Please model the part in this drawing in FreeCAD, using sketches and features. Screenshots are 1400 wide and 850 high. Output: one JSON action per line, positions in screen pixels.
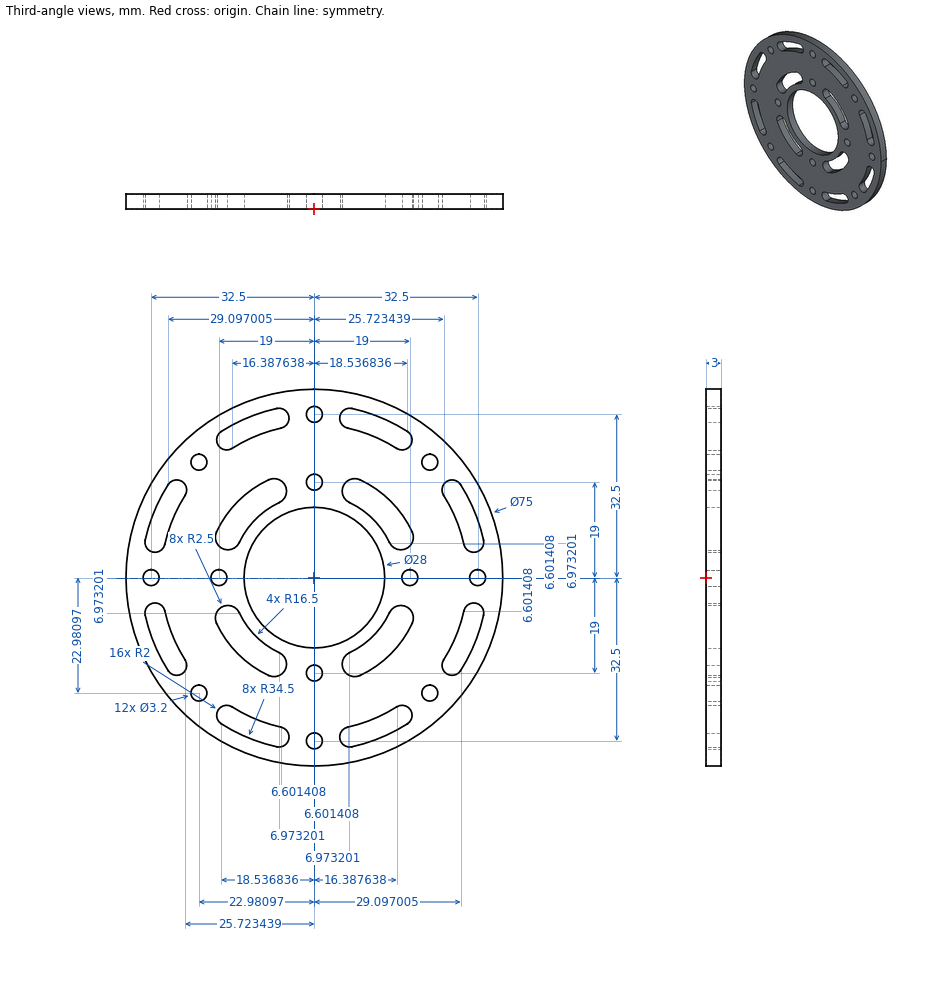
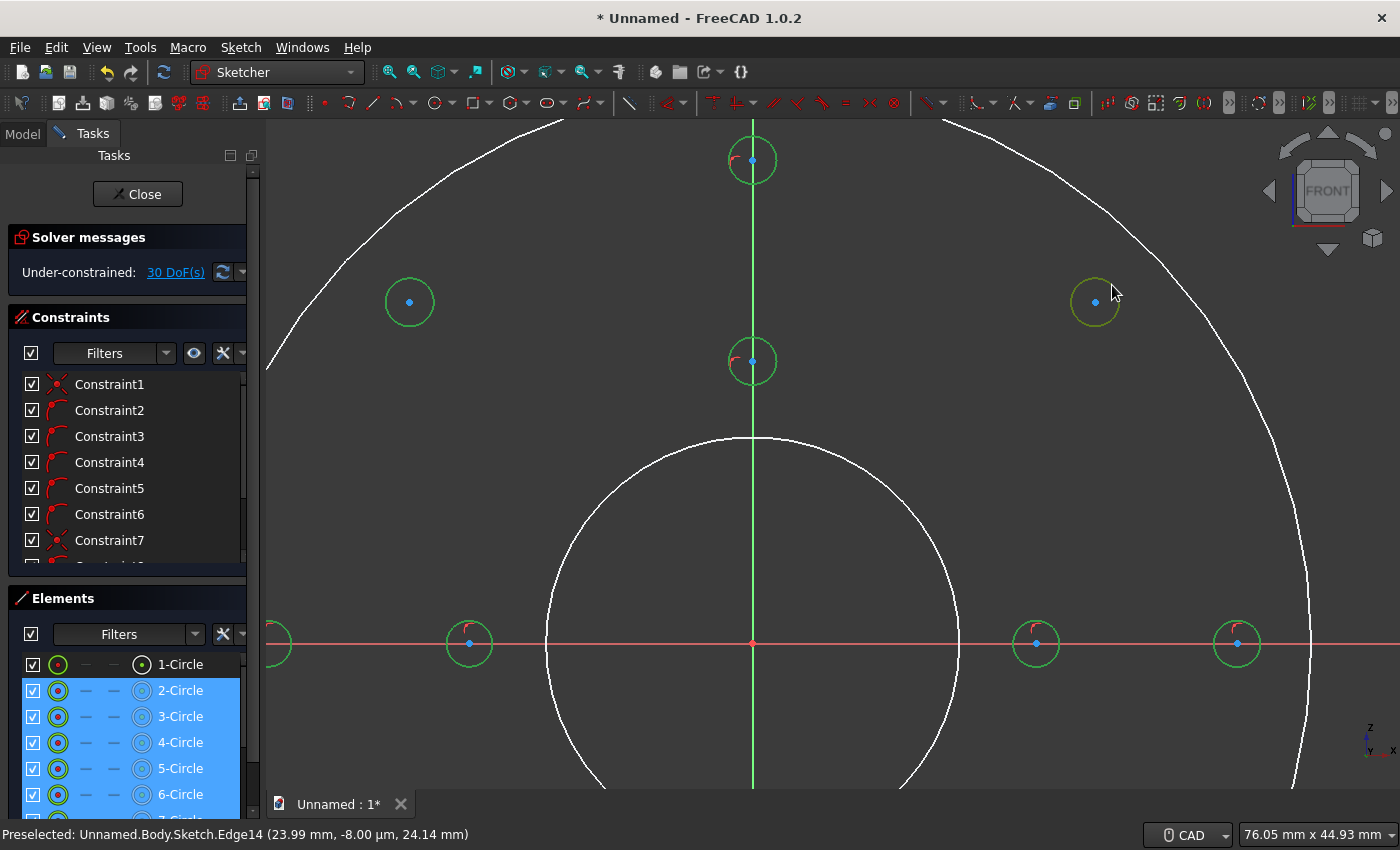
{"action": "left_click", "coordinate": [846, 104]}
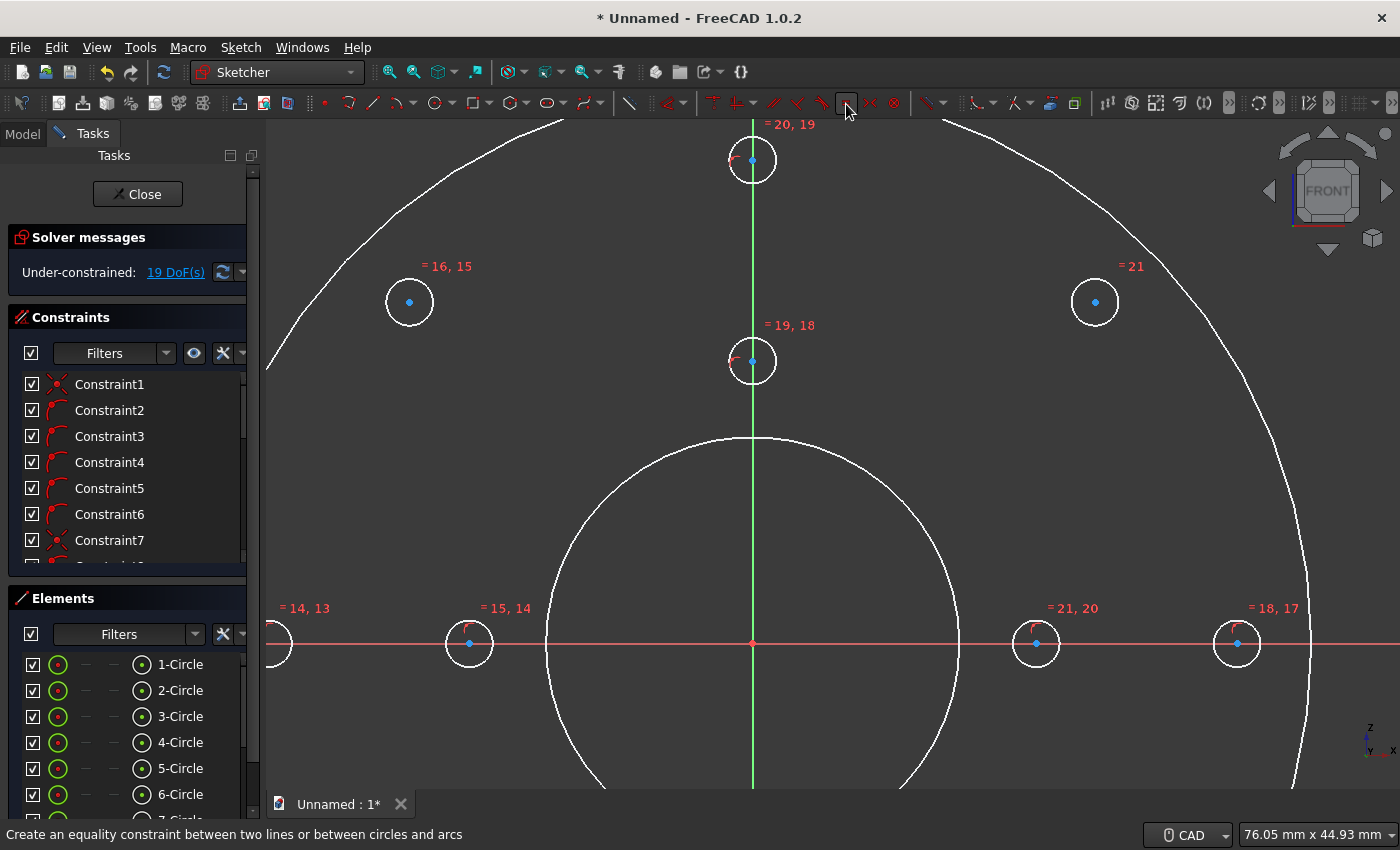
{"action": "scroll", "coordinate": [771, 344], "scroll_direction": "down", "scroll_amount": 5}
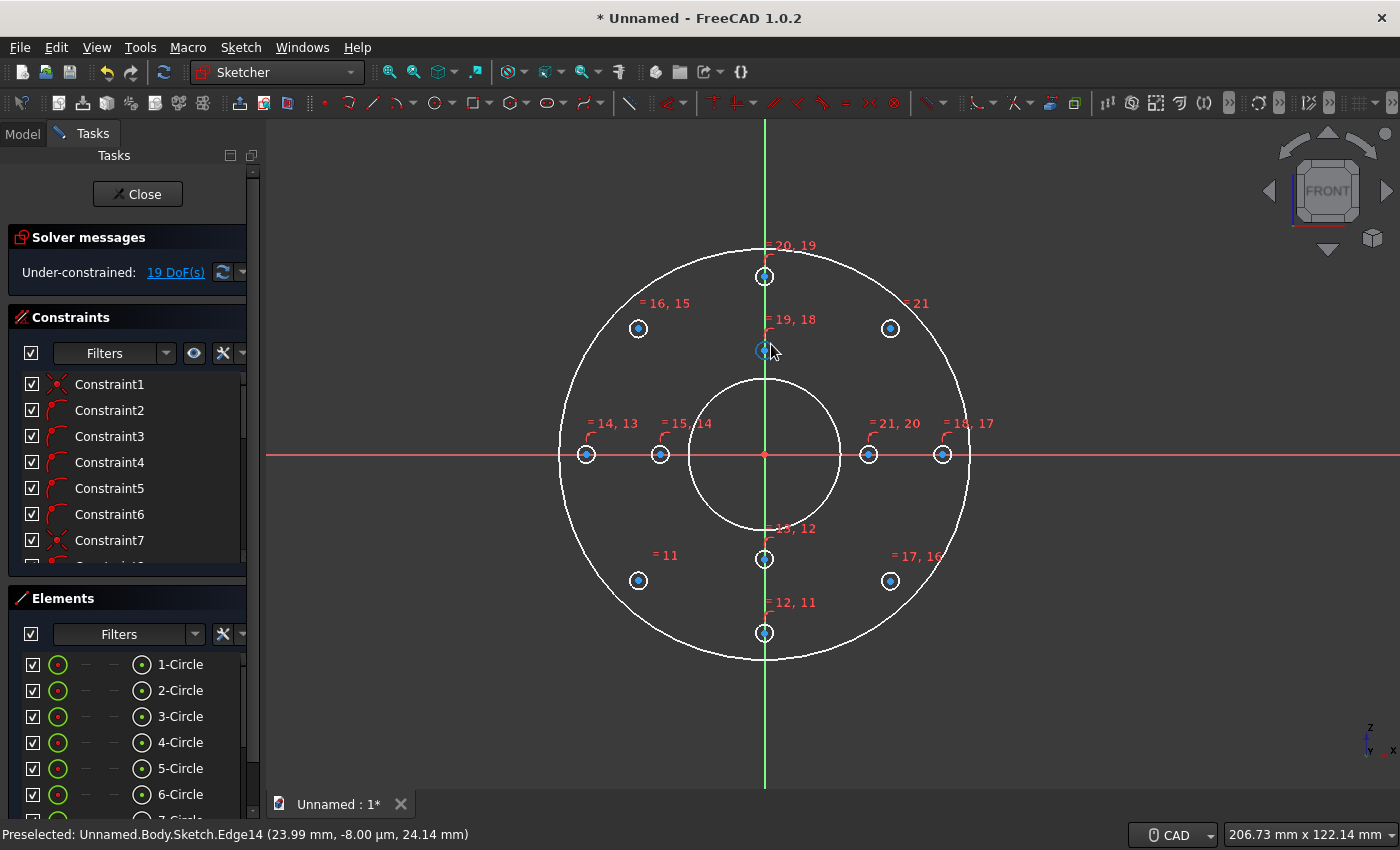
{"action": "left_click", "coordinate": [639, 581]}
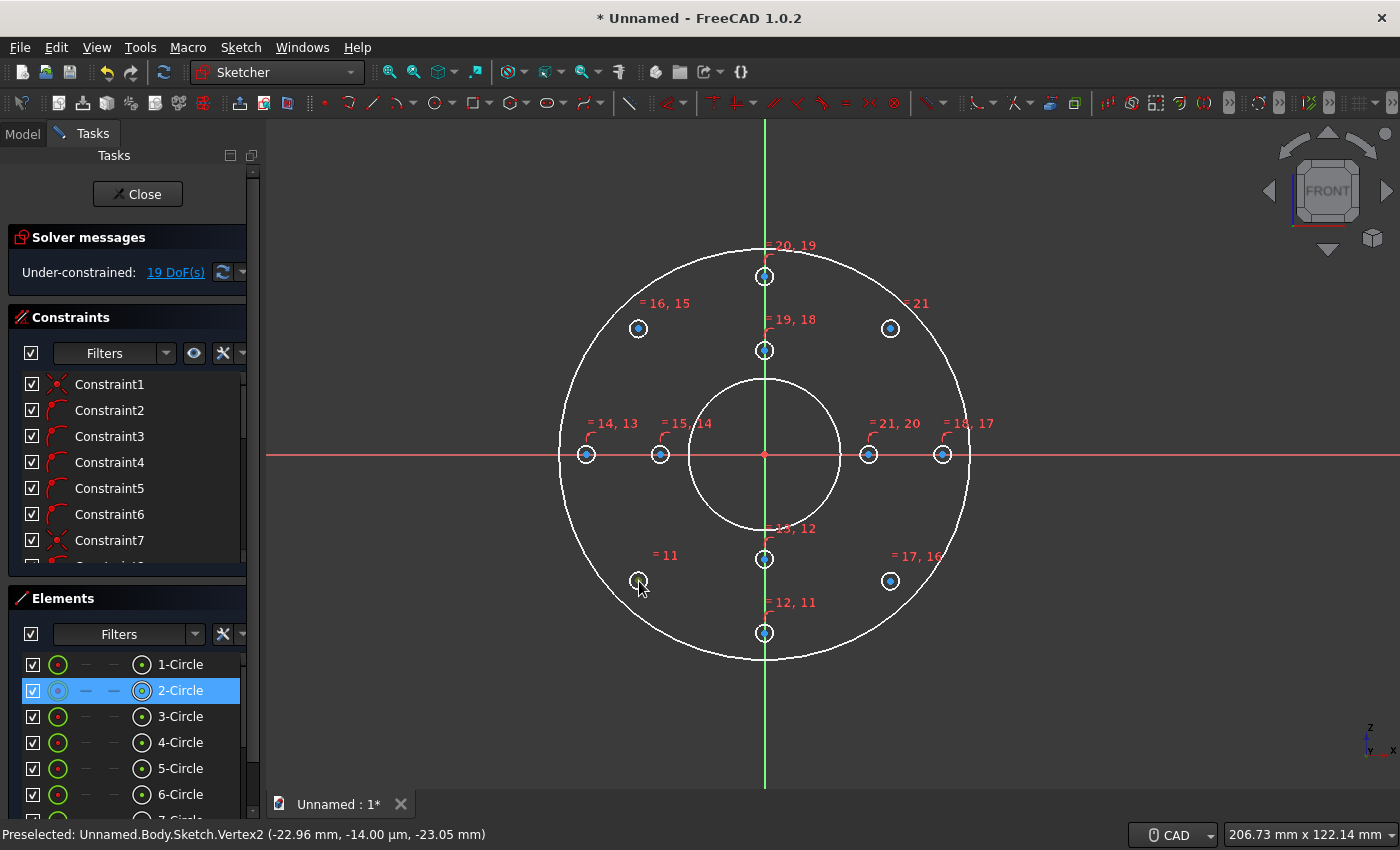
{"action": "left_click", "coordinate": [638, 329]}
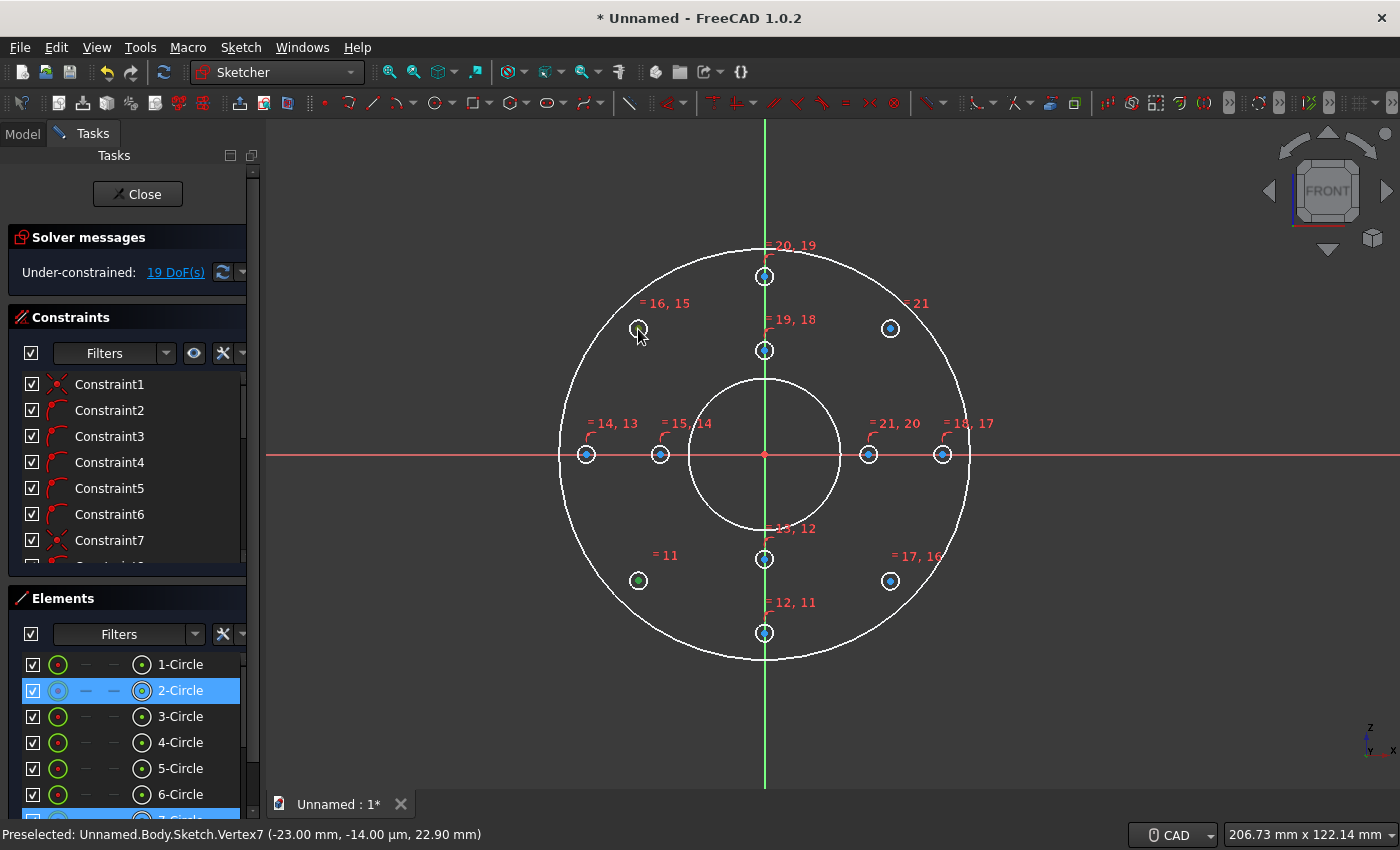
{"action": "left_click", "coordinate": [756, 104]}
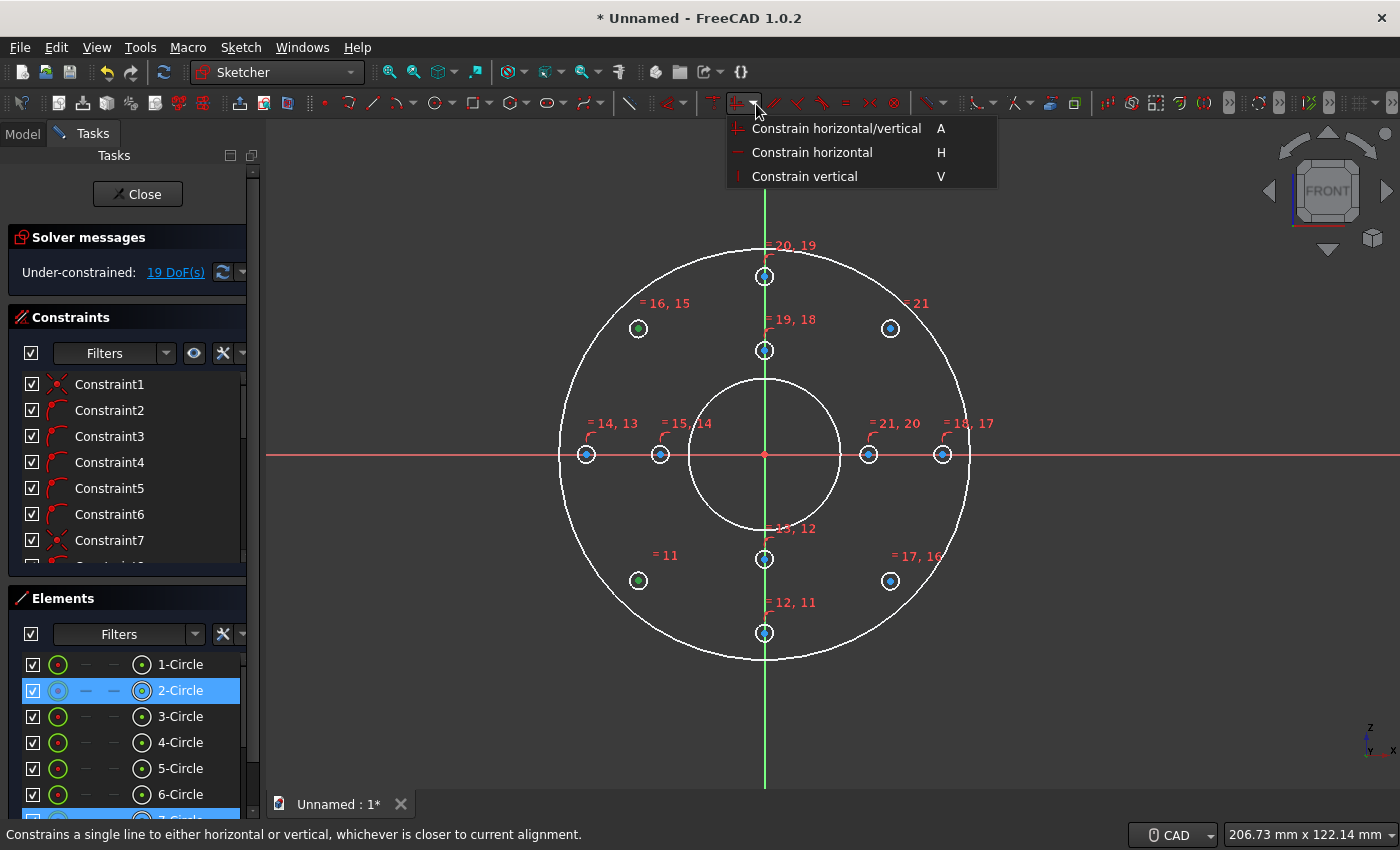
{"action": "left_click", "coordinate": [862, 176]}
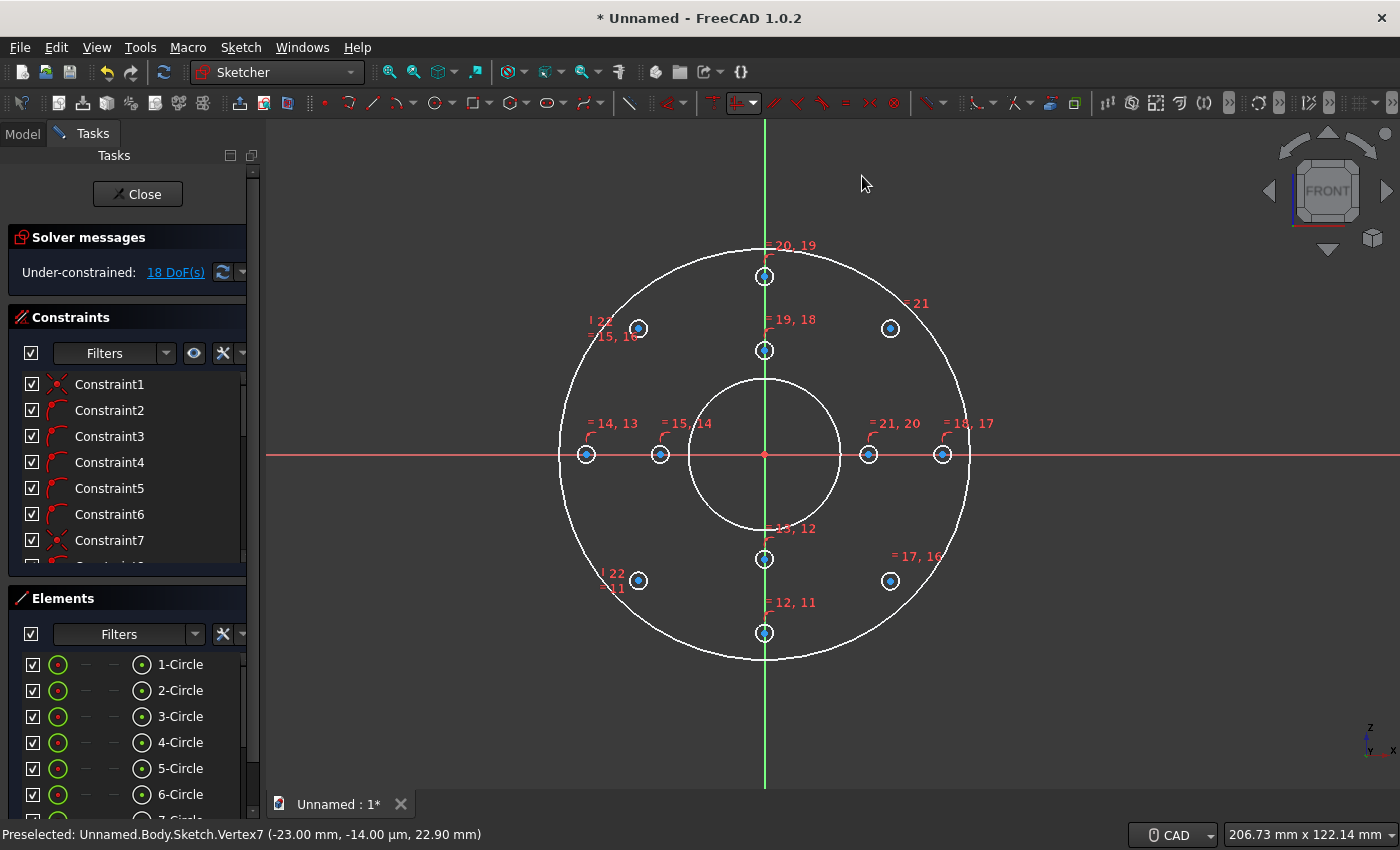
{"action": "left_click", "coordinate": [639, 581]}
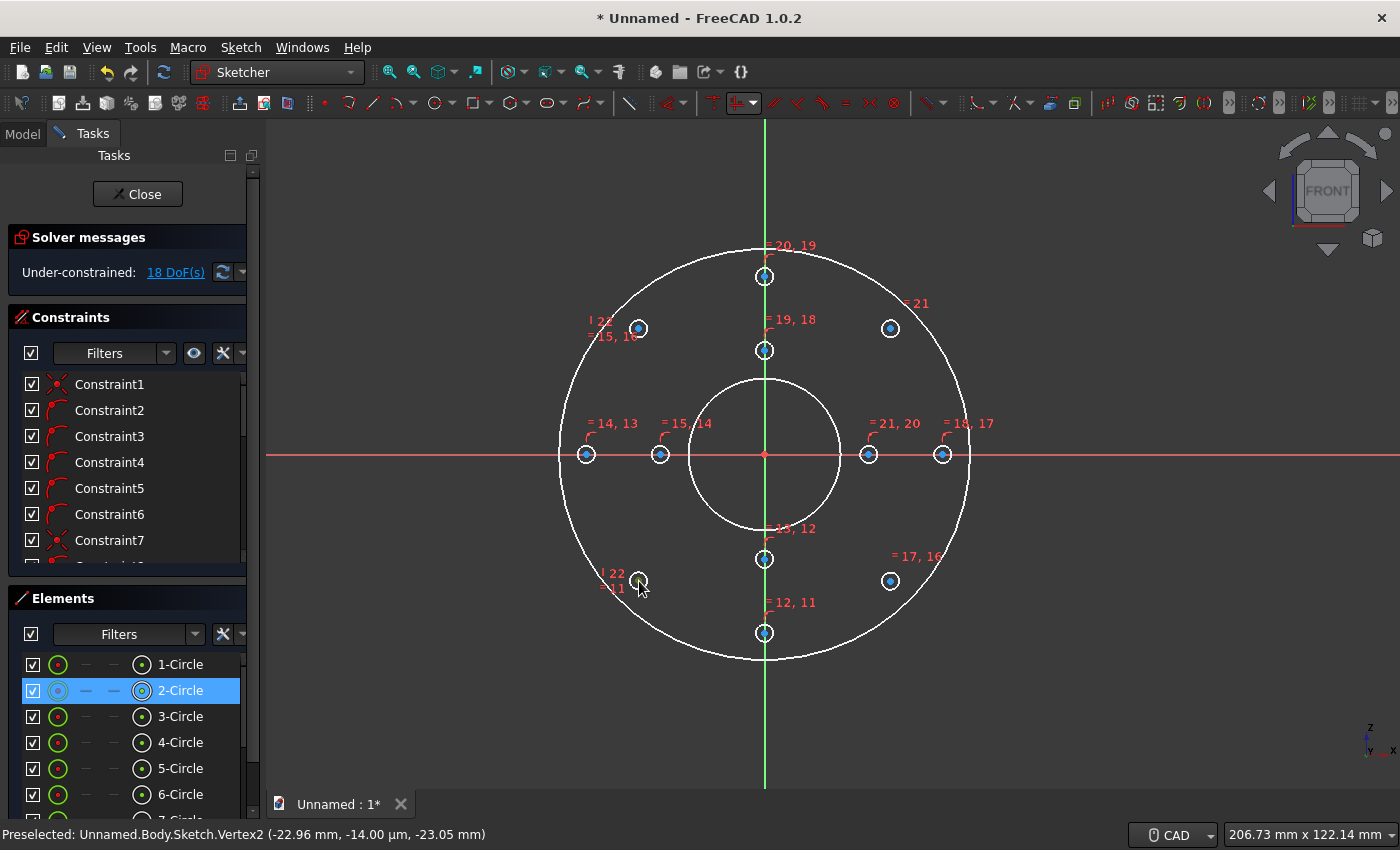
{"action": "left_click", "coordinate": [891, 581]}